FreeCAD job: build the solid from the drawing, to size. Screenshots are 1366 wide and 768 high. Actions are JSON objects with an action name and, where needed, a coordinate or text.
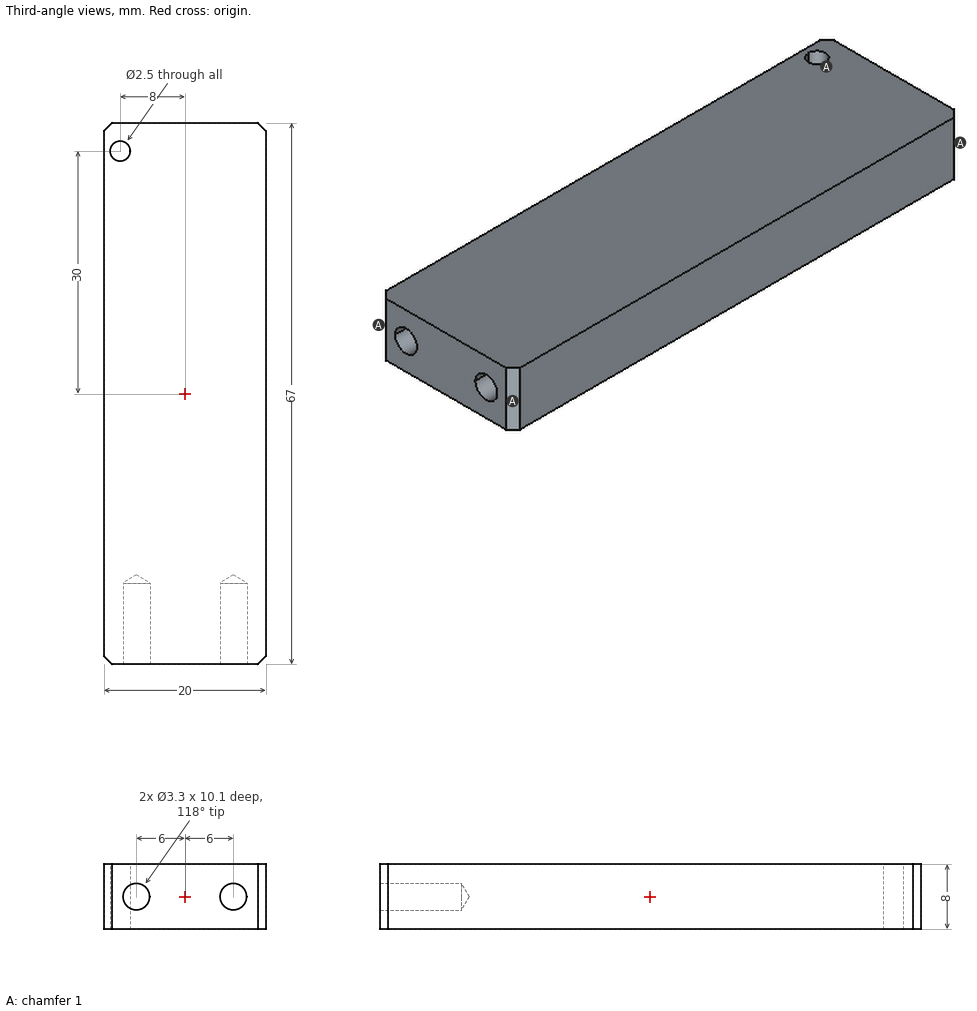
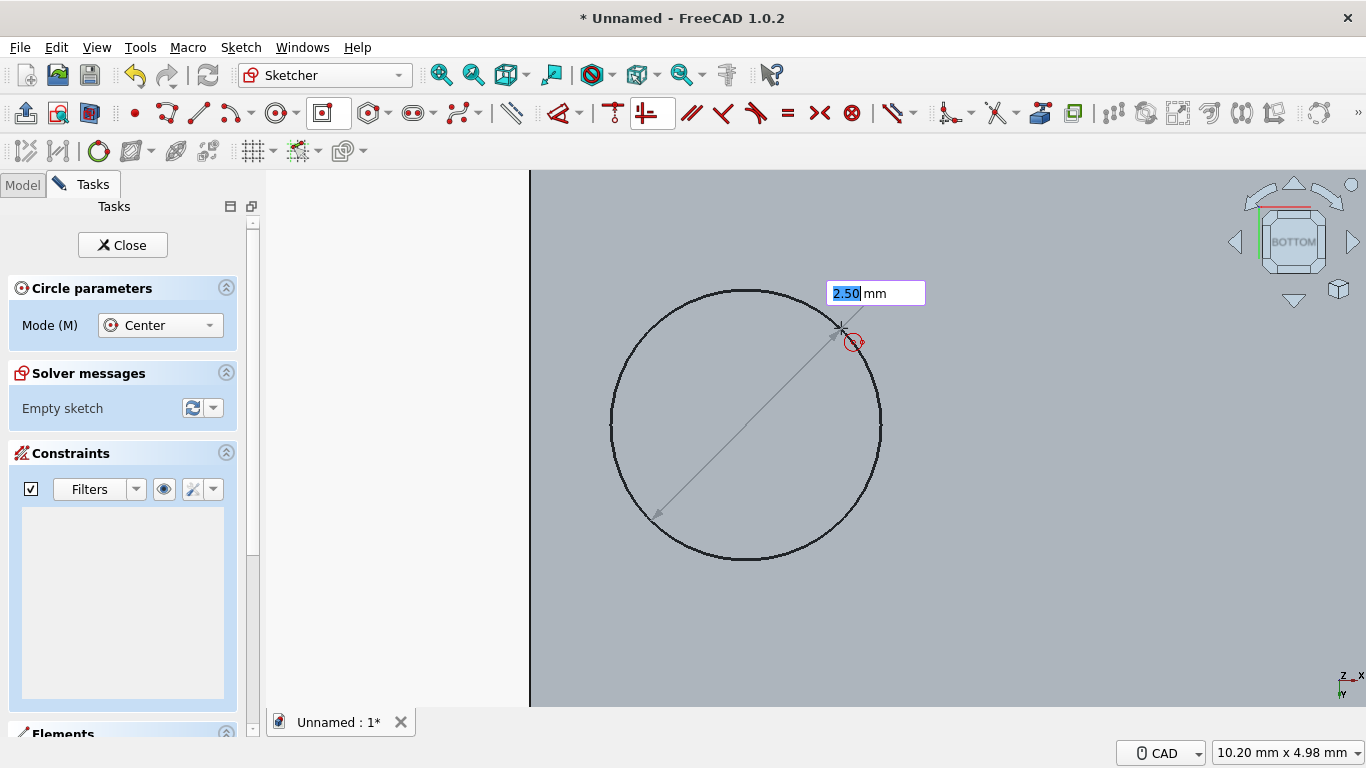
{"action": "type", "text": "2.5"}
{"action": "key", "text": "Return"}
{"action": "key", "text": "Escape"}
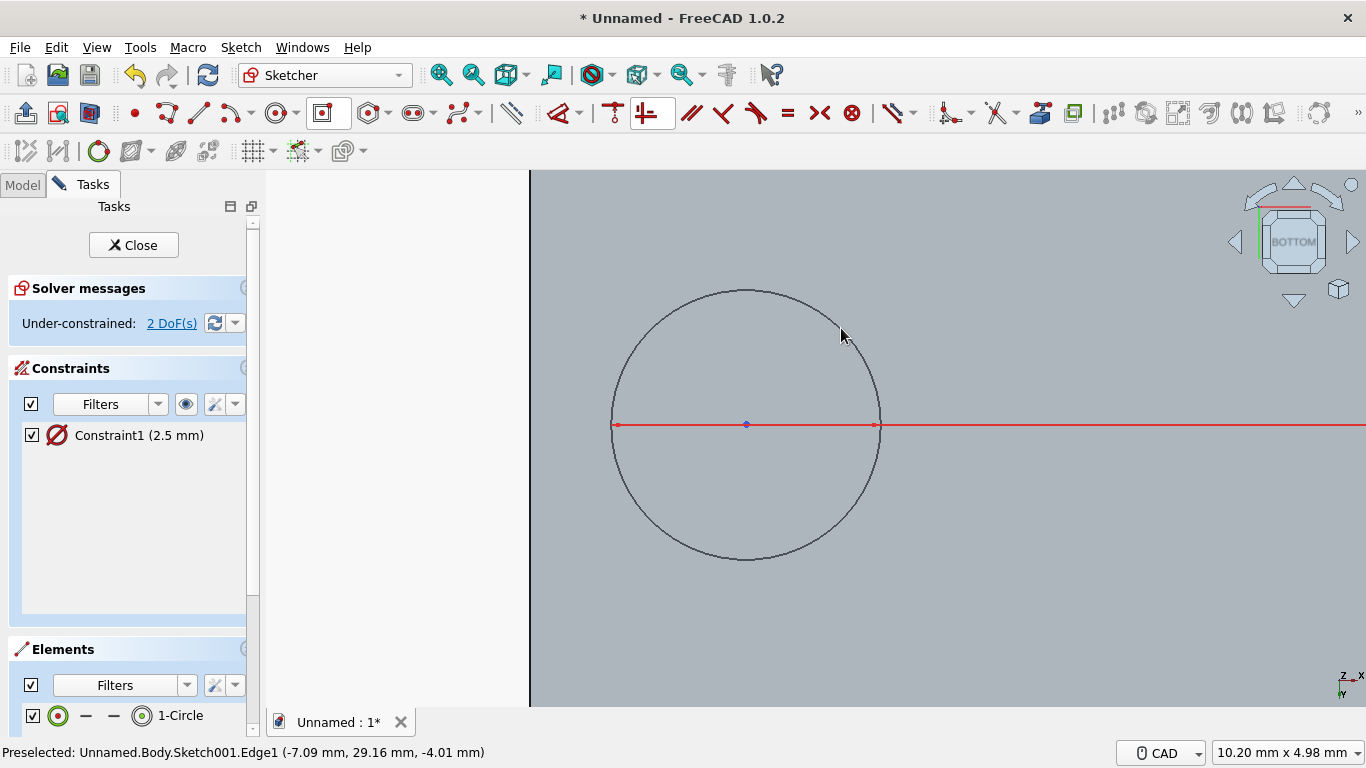
{"action": "key", "text": "d"}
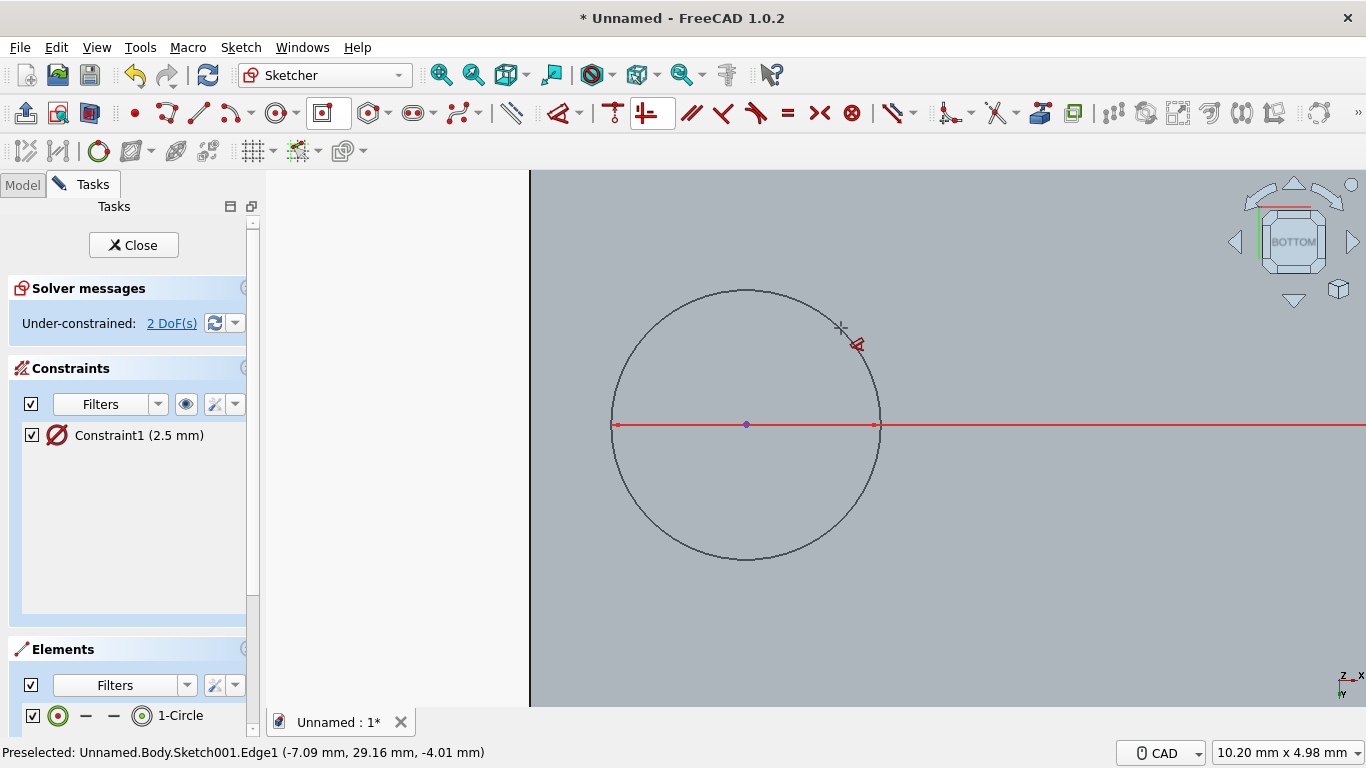
{"action": "left_click", "coordinate": [746, 425]}
{"action": "left_click", "coordinate": [974, 459]}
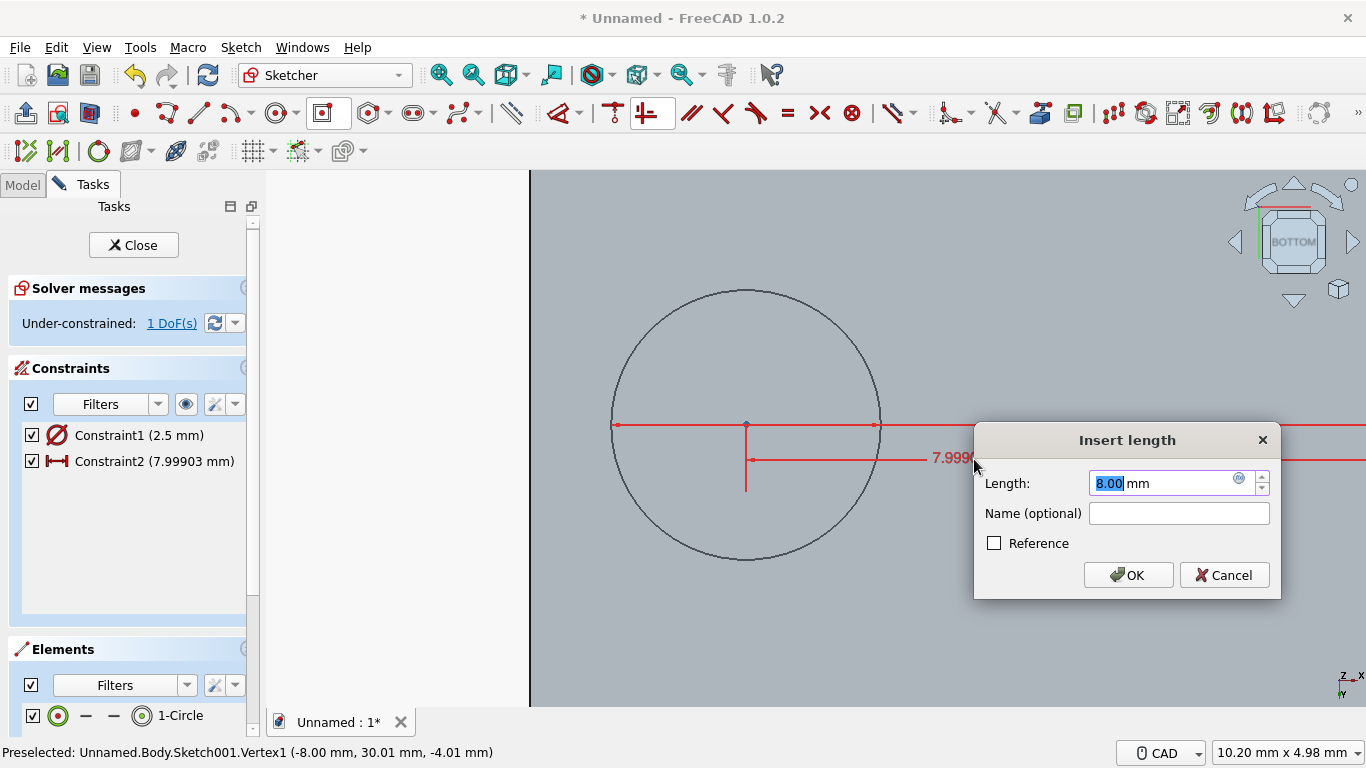
{"action": "type", "text": "8"}
{"action": "key", "text": "Return"}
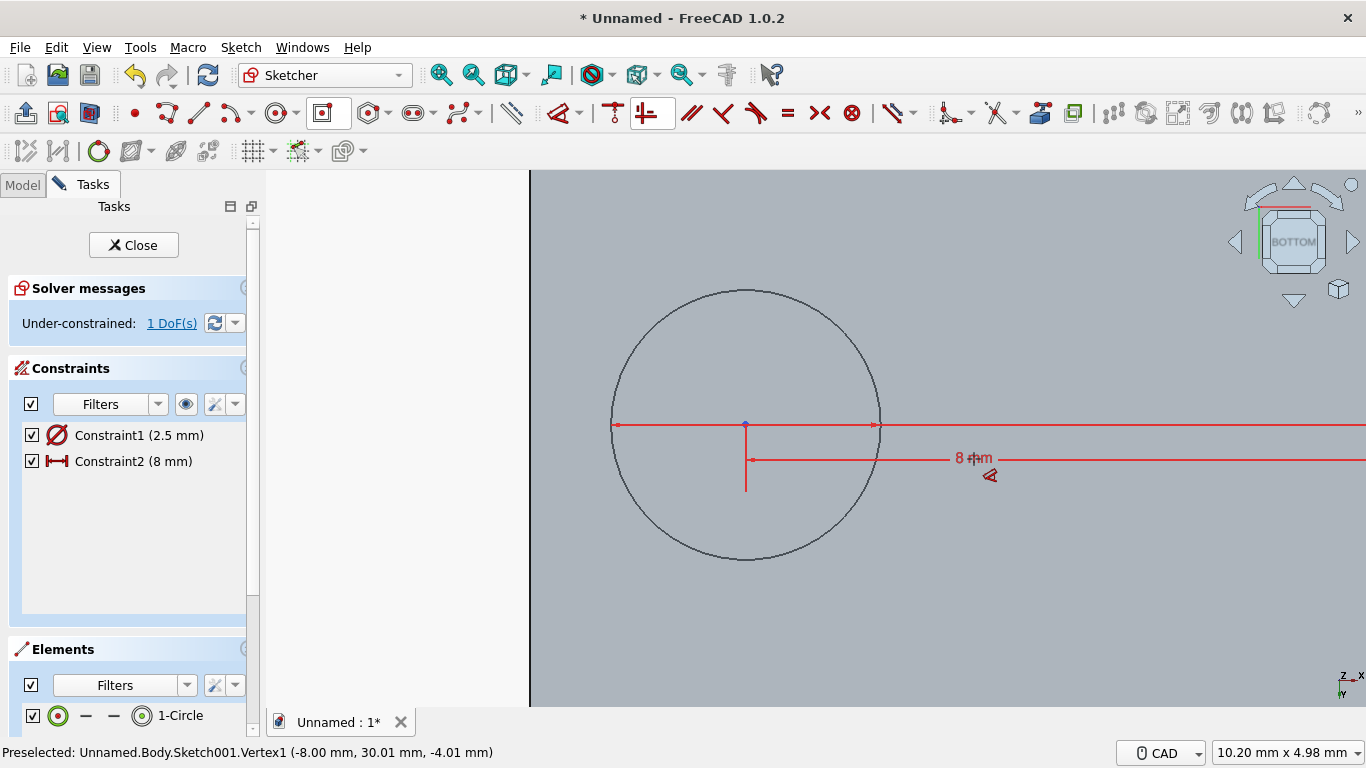
{"action": "left_click", "coordinate": [746, 425]}
{"action": "left_click", "coordinate": [712, 311]}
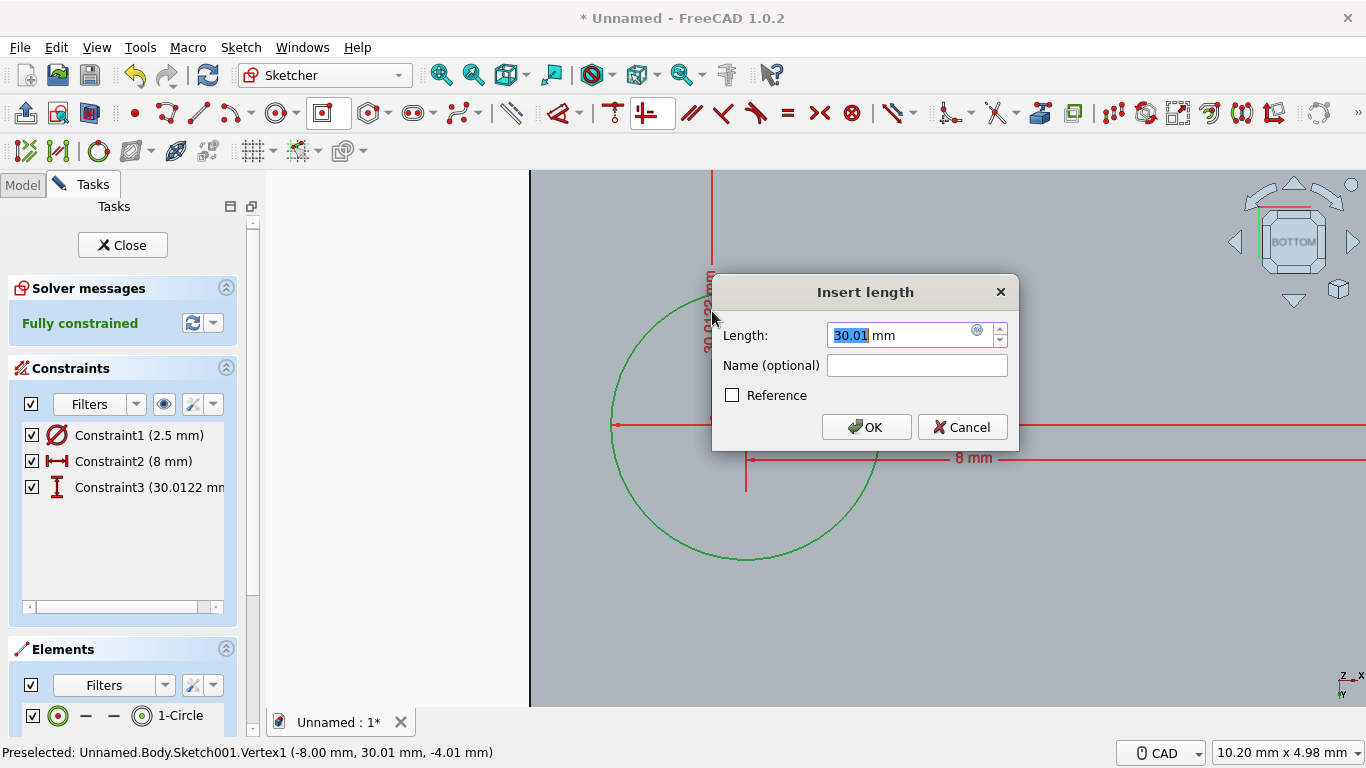
{"action": "type", "text": "30"}
{"action": "key", "text": "Return"}
{"action": "key", "text": "Escape"}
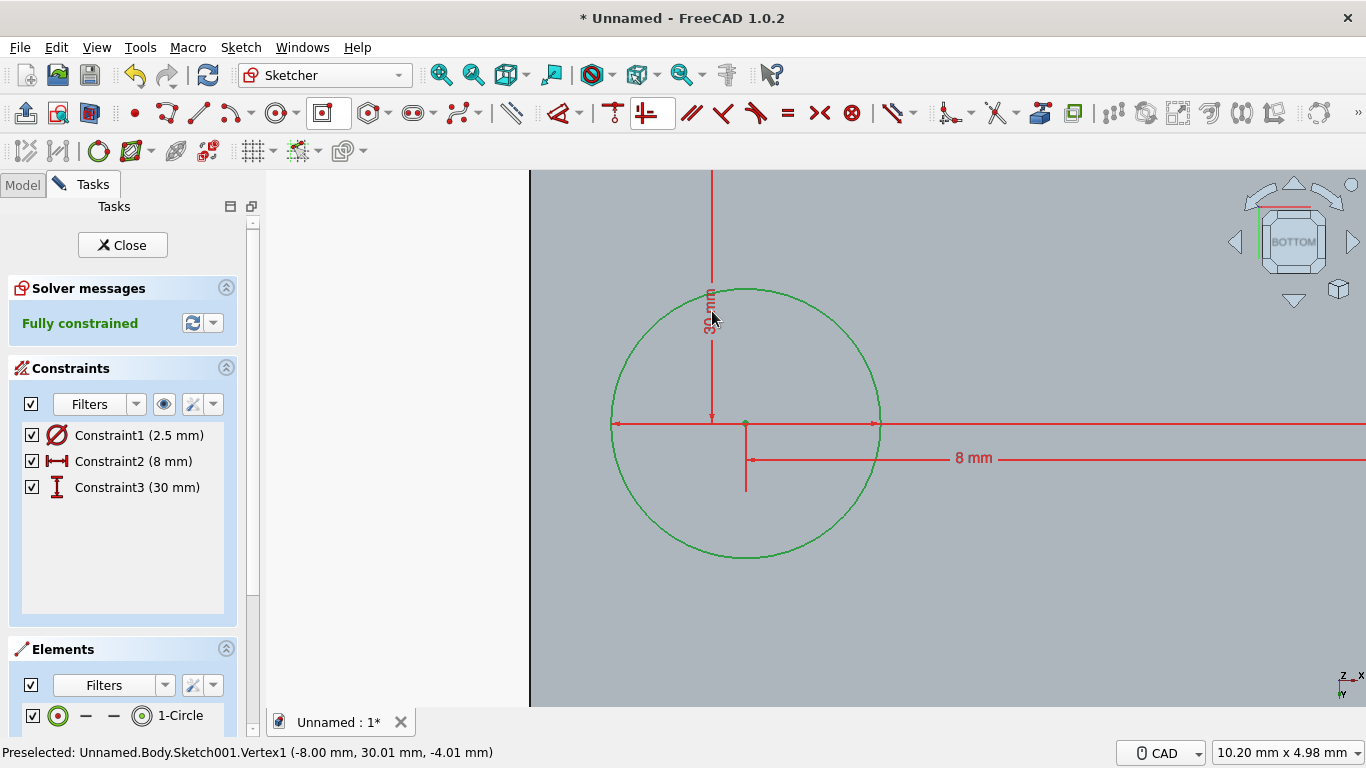
{"action": "left_click", "coordinate": [123, 245]}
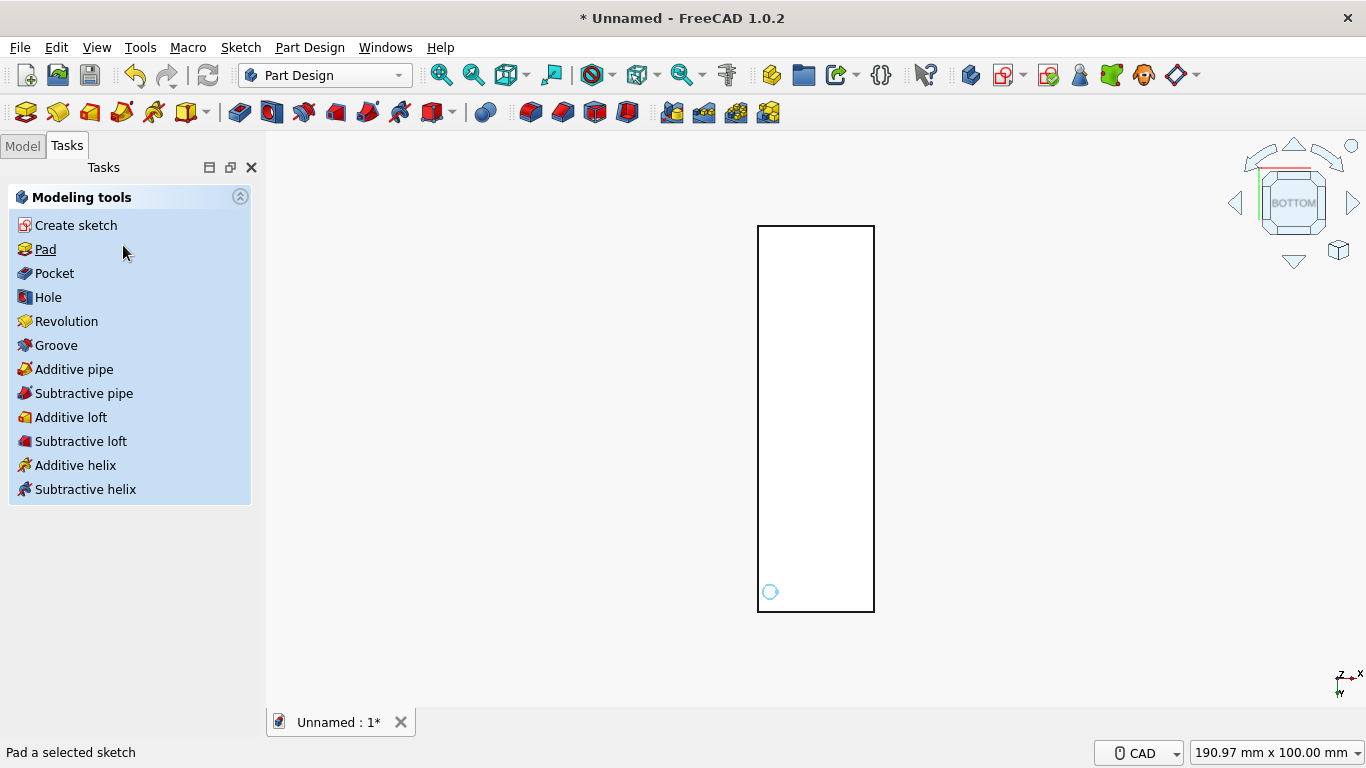
{"action": "left_click", "coordinate": [272, 112]}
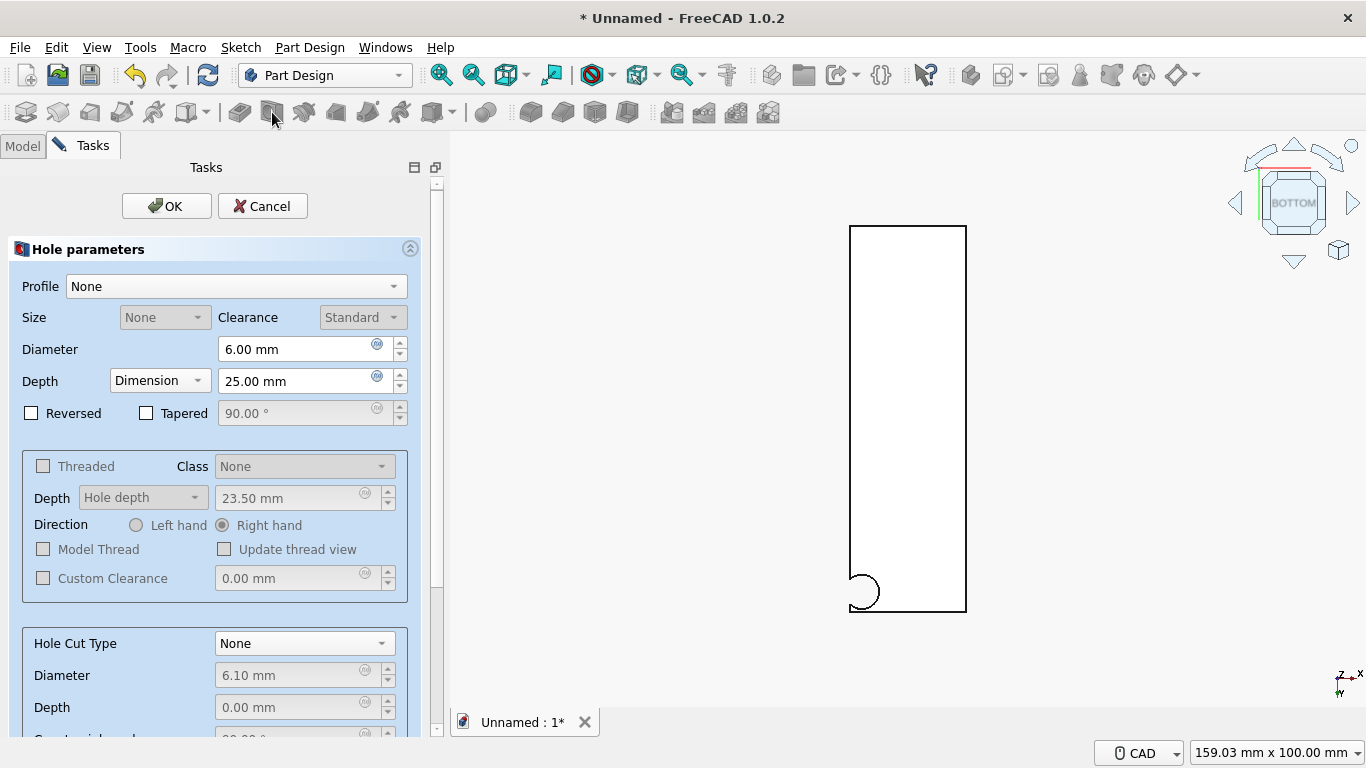
{"action": "triple_click", "coordinate": [305, 349]}